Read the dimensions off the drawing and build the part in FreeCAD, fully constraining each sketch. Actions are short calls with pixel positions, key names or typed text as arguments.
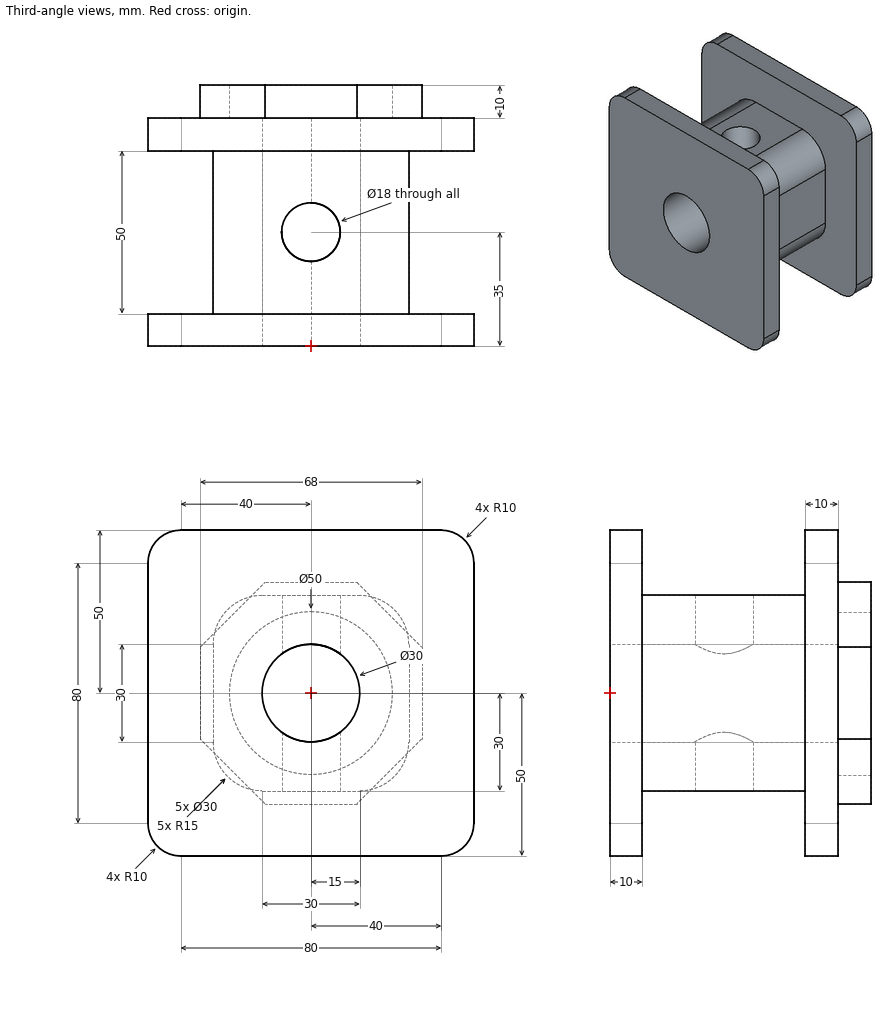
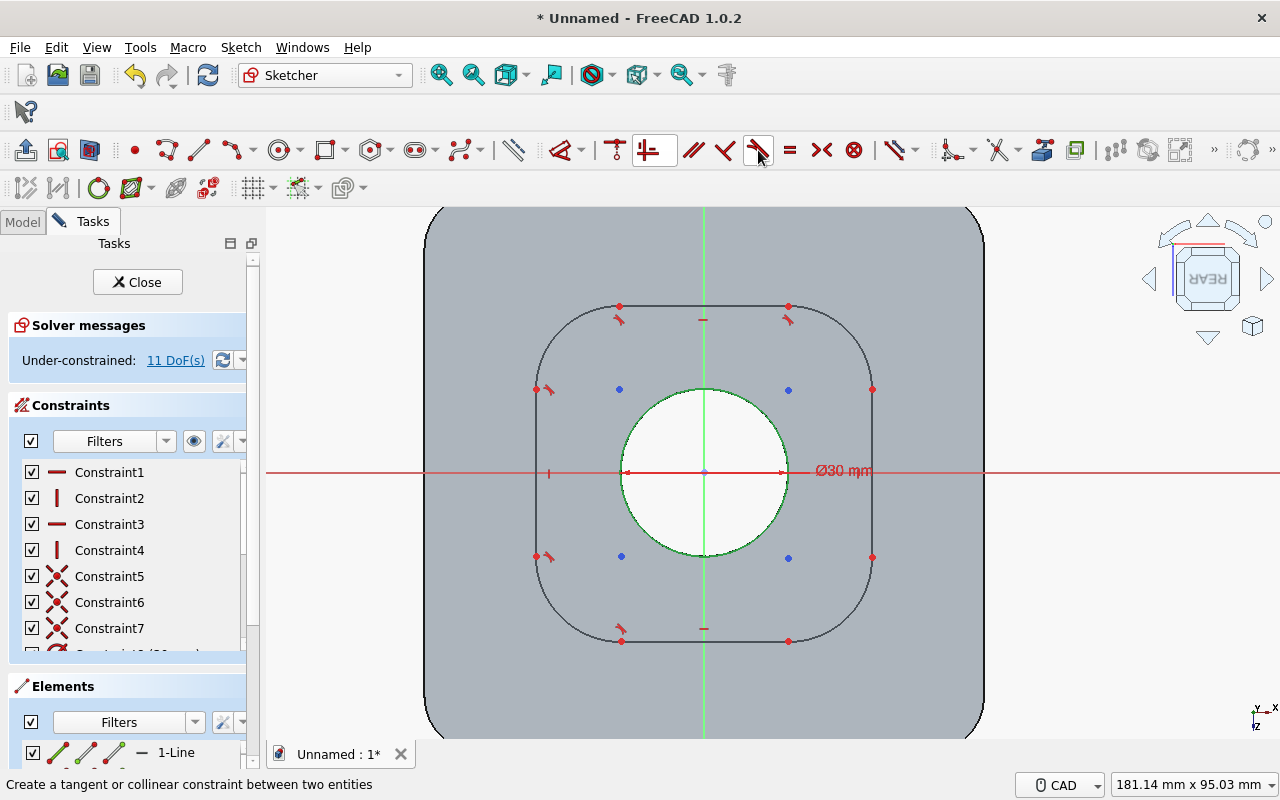
click(671, 642)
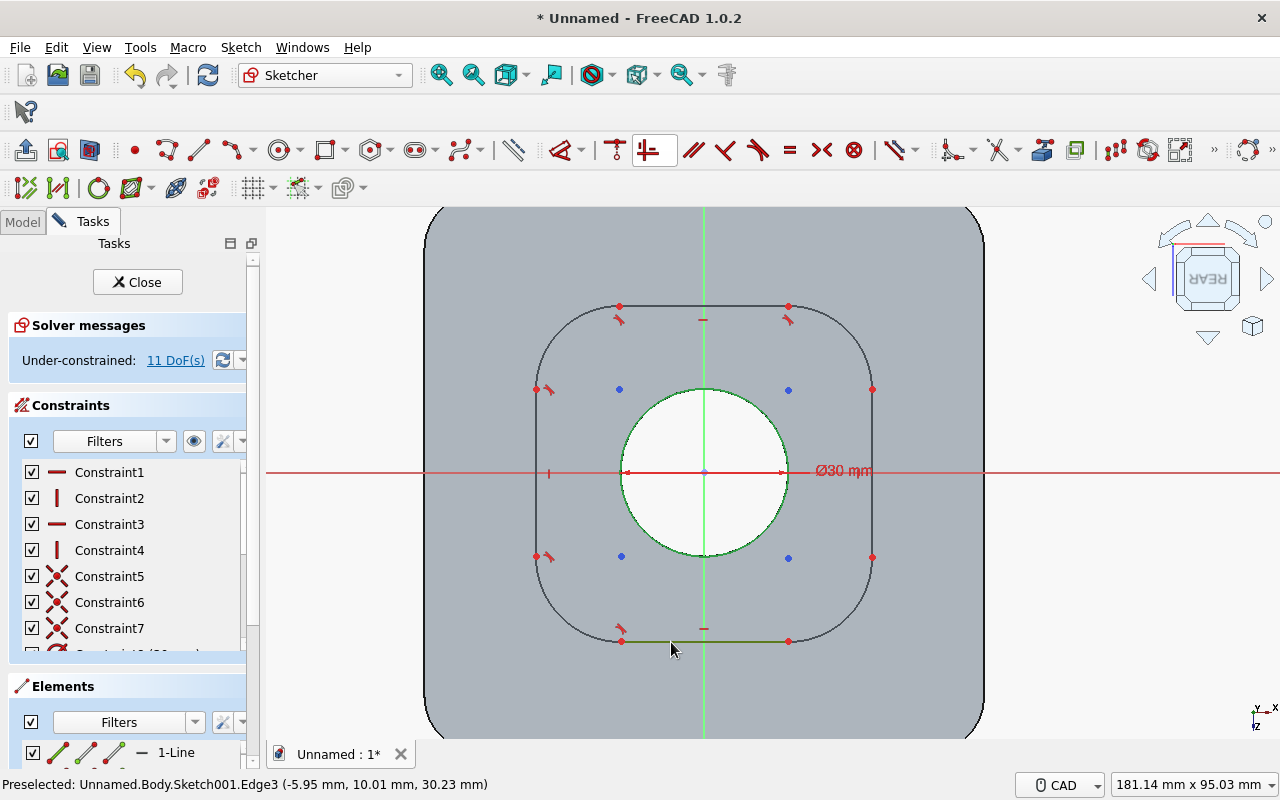
click(826, 633)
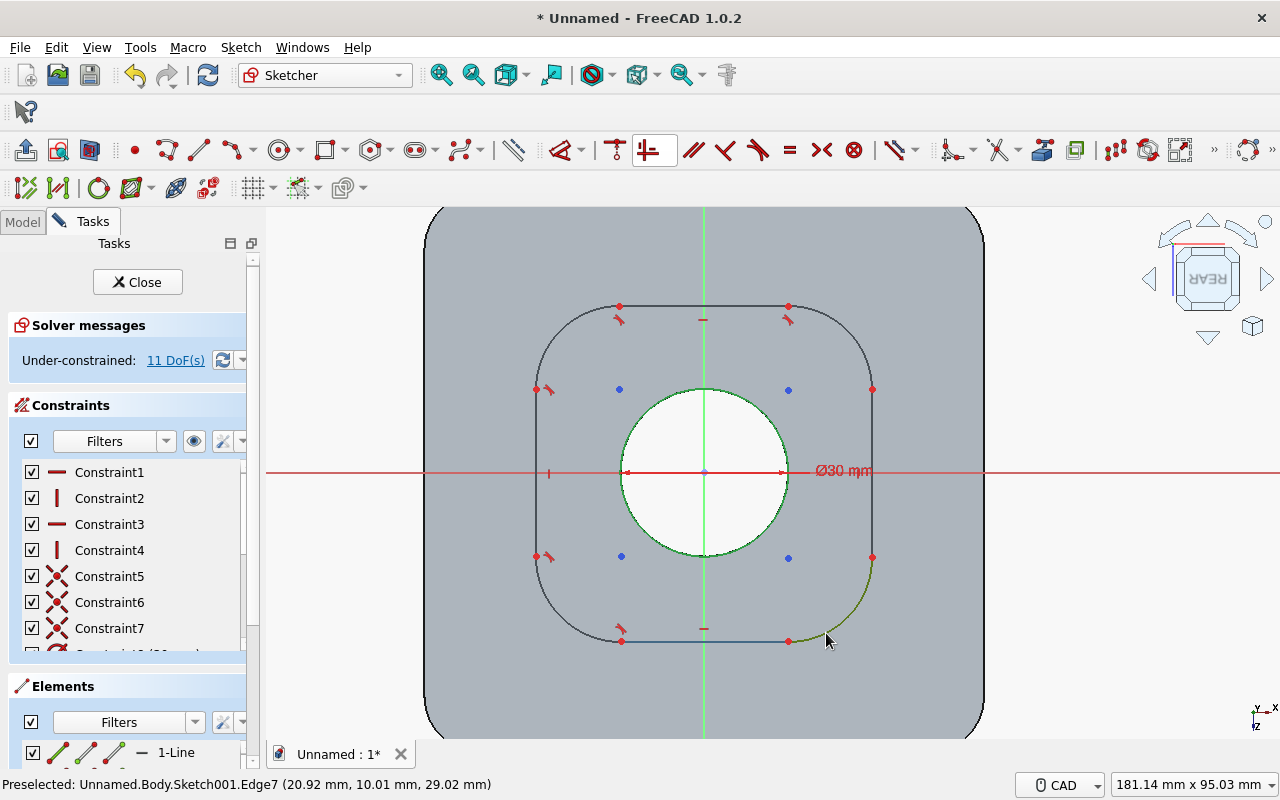
click(758, 150)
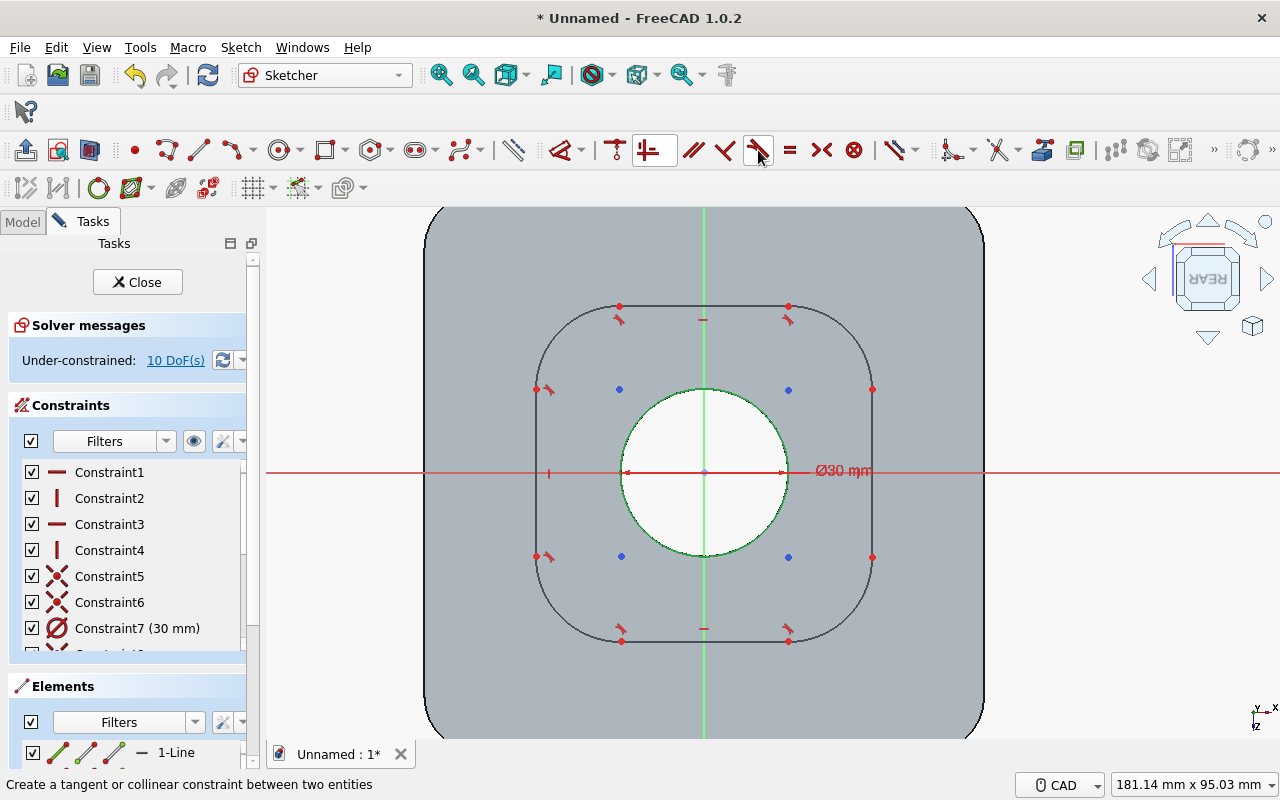
click(872, 508)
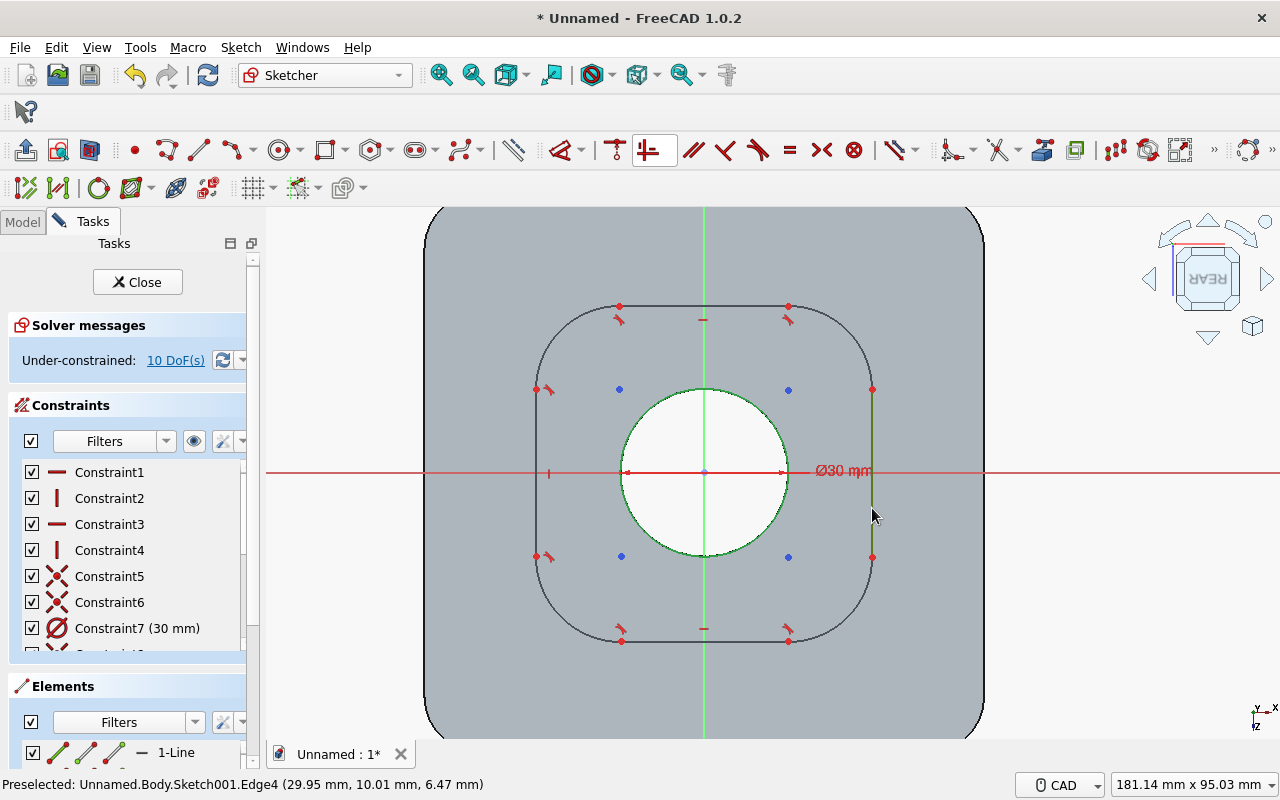
click(826, 633)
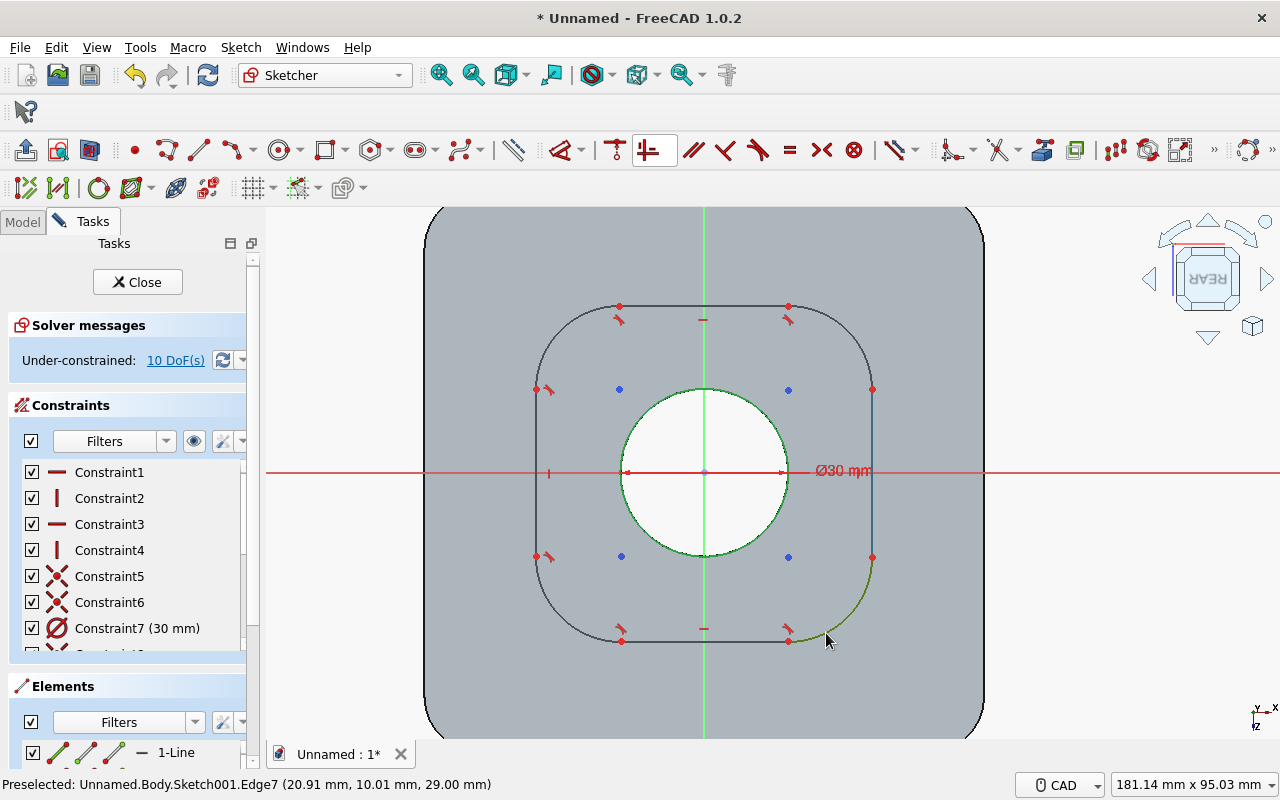
click(758, 150)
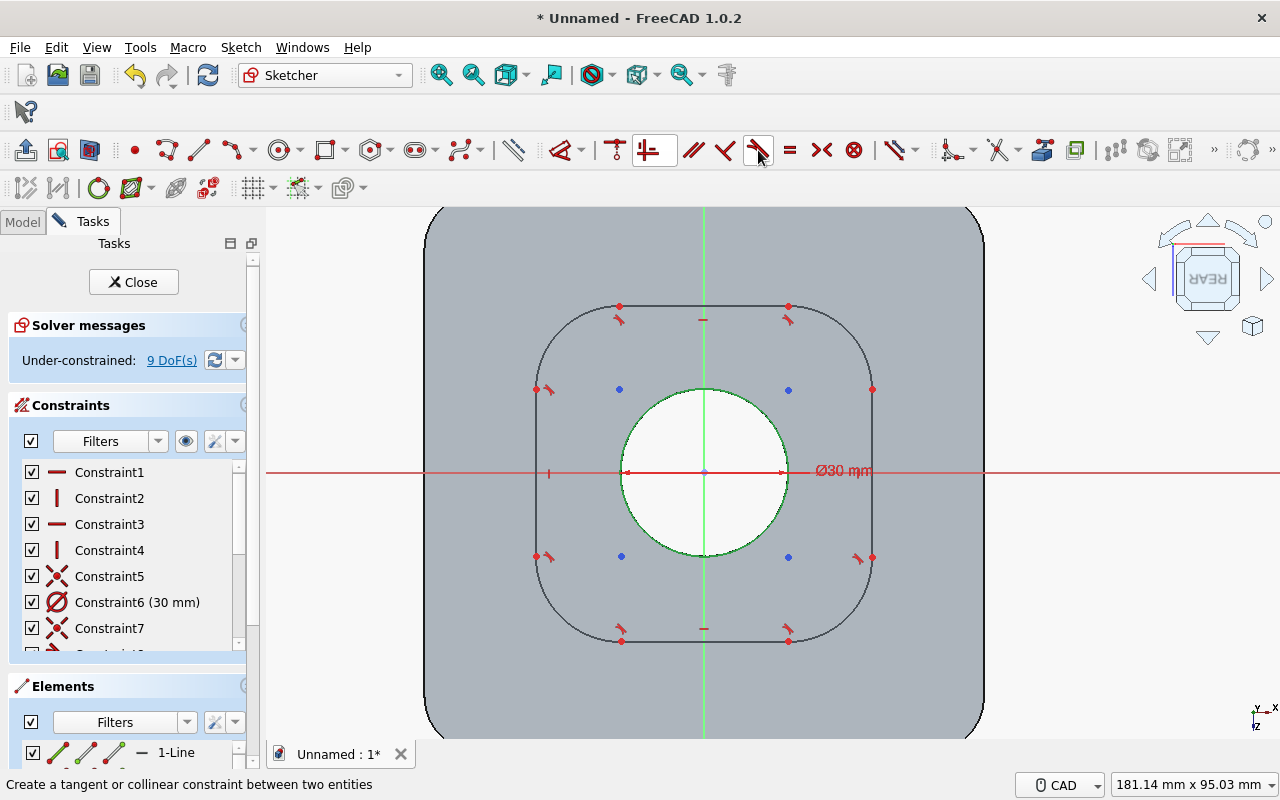
click(872, 508)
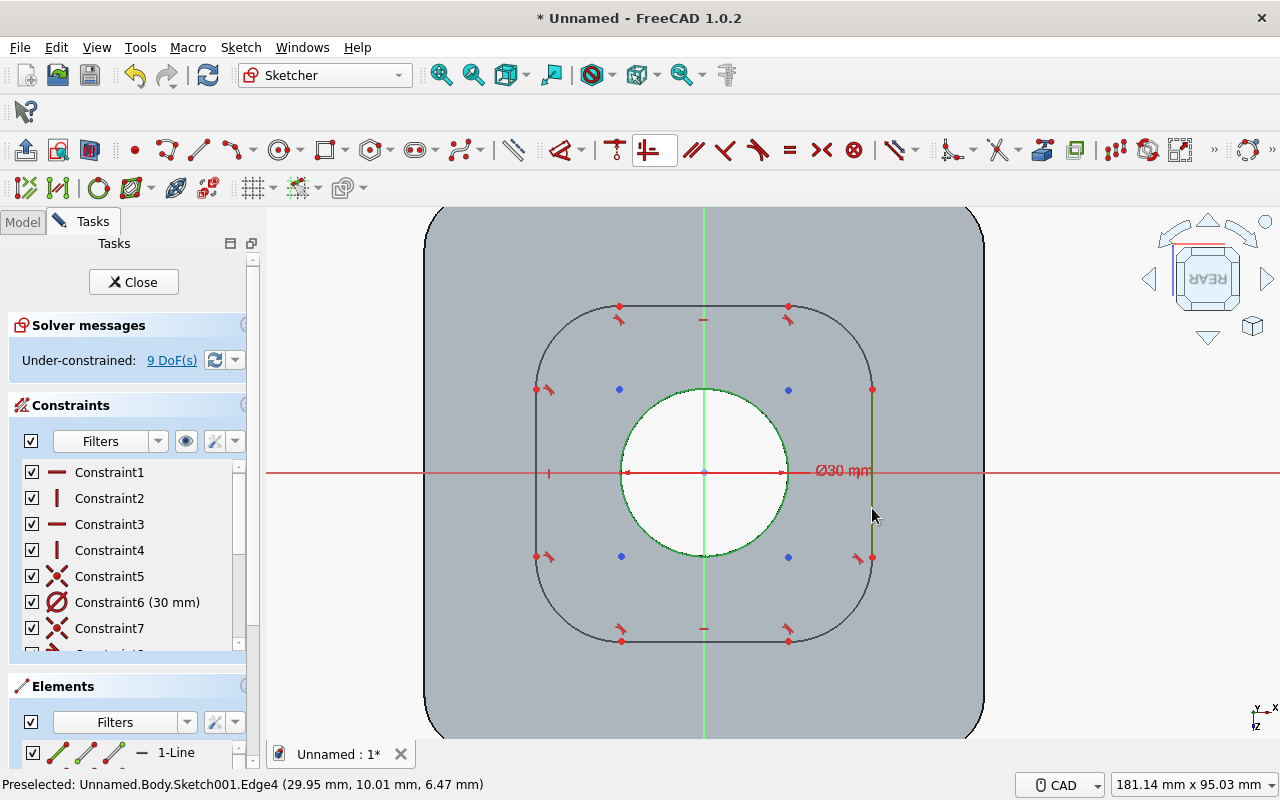
click(863, 352)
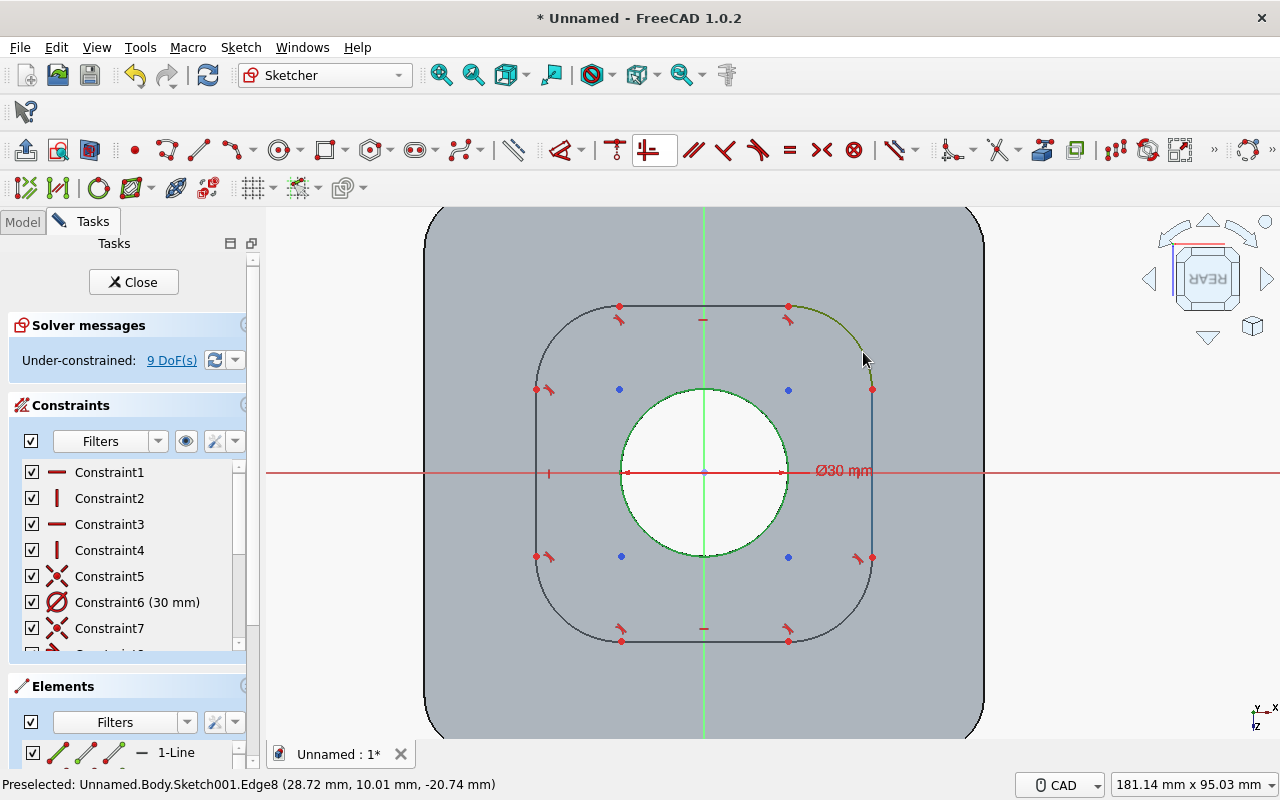
click(758, 150)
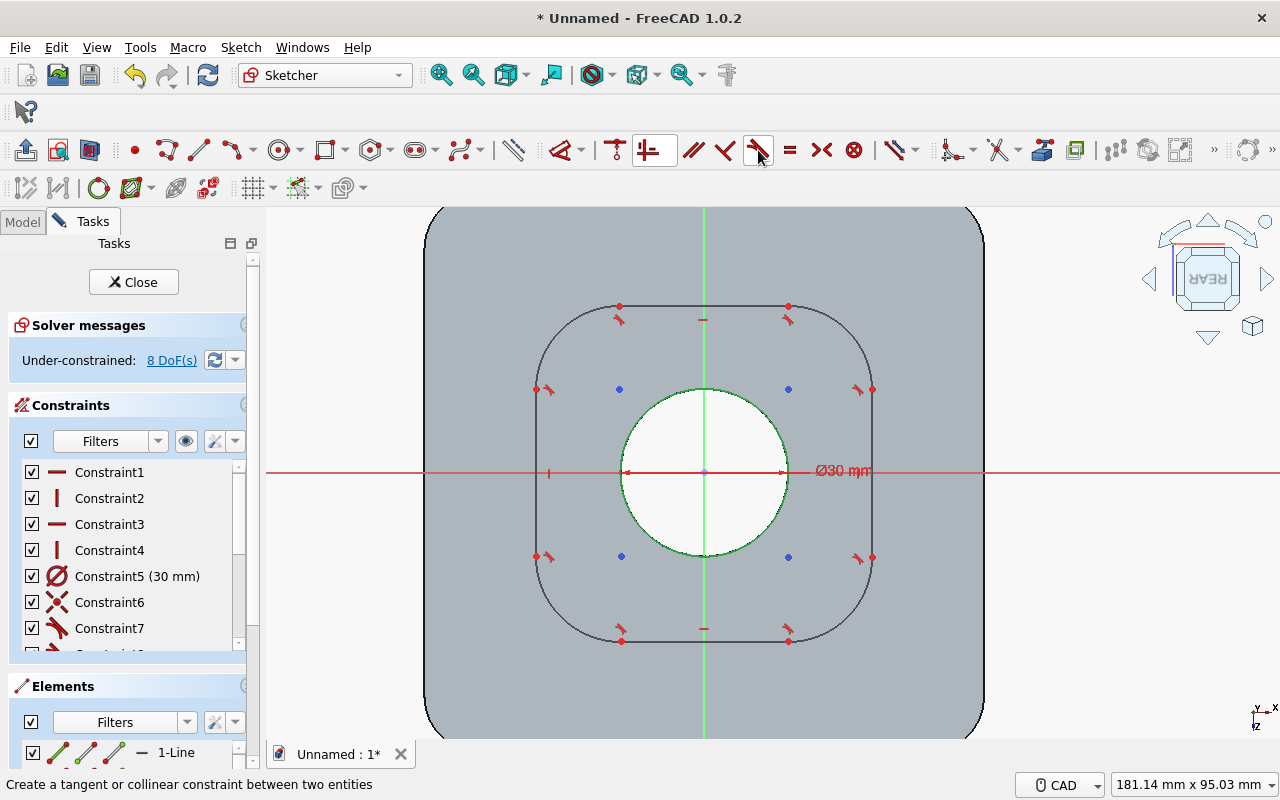
click(582, 315)